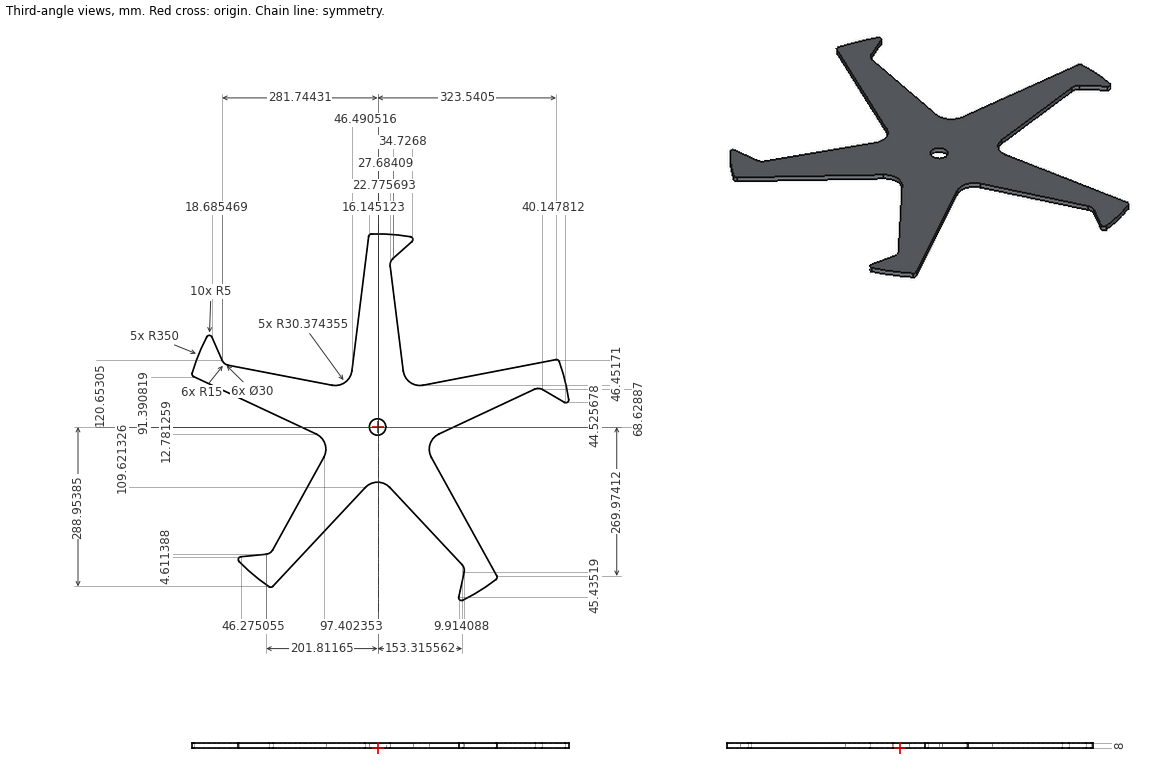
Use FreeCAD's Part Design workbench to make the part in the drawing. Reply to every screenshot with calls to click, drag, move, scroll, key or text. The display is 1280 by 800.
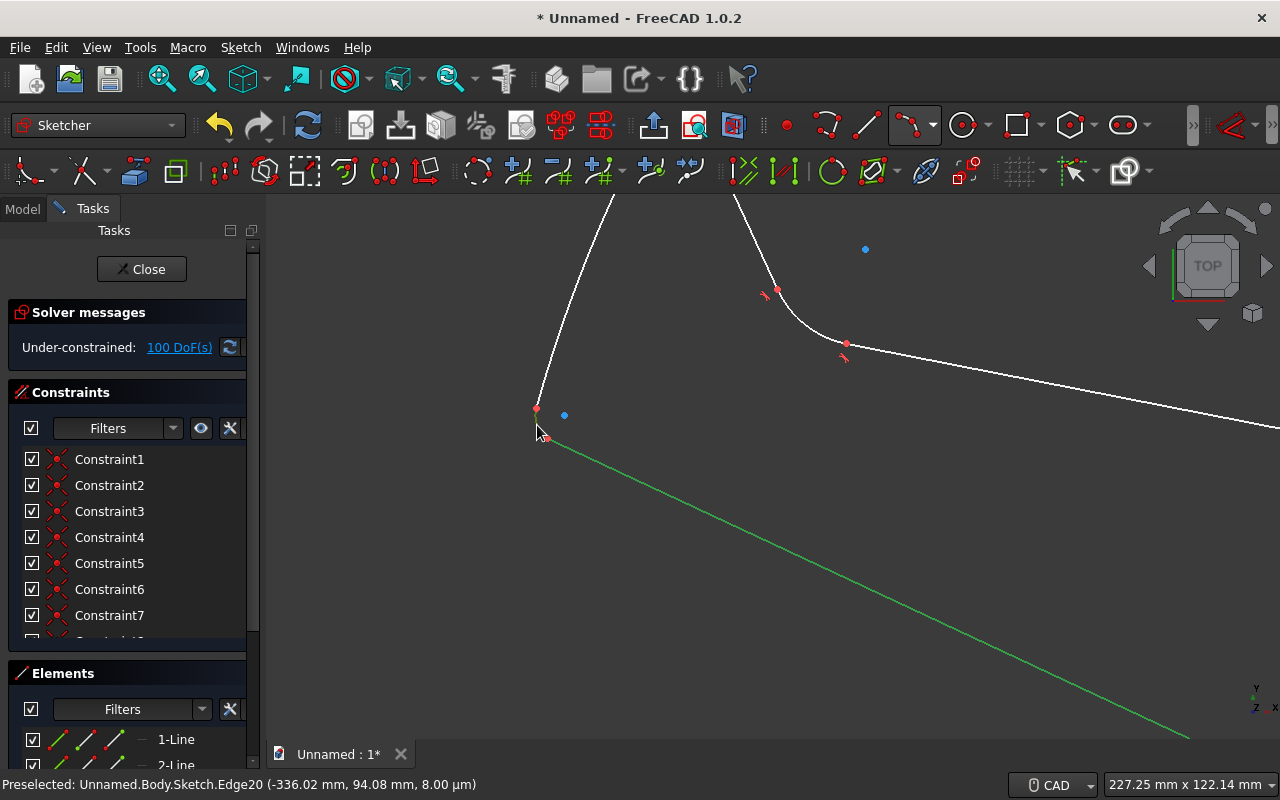
key(t)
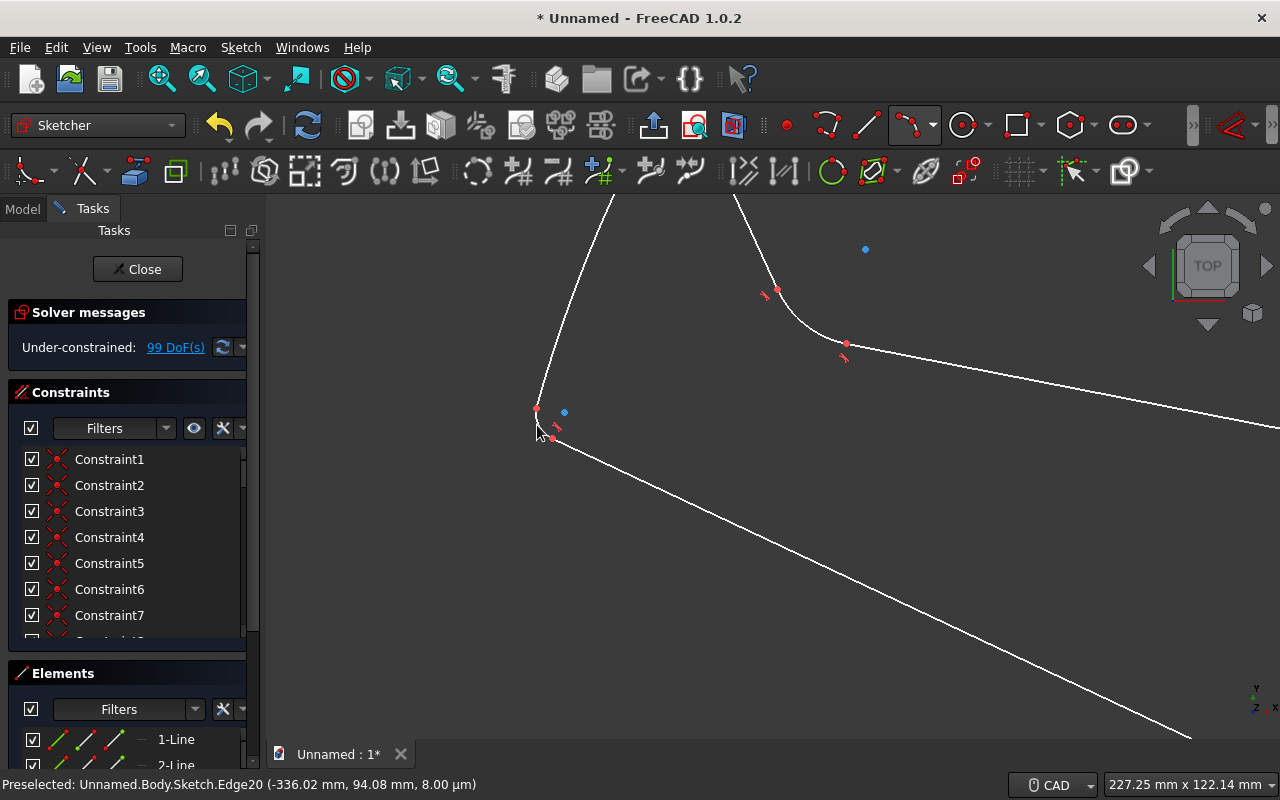
scroll(536, 430, down, 11)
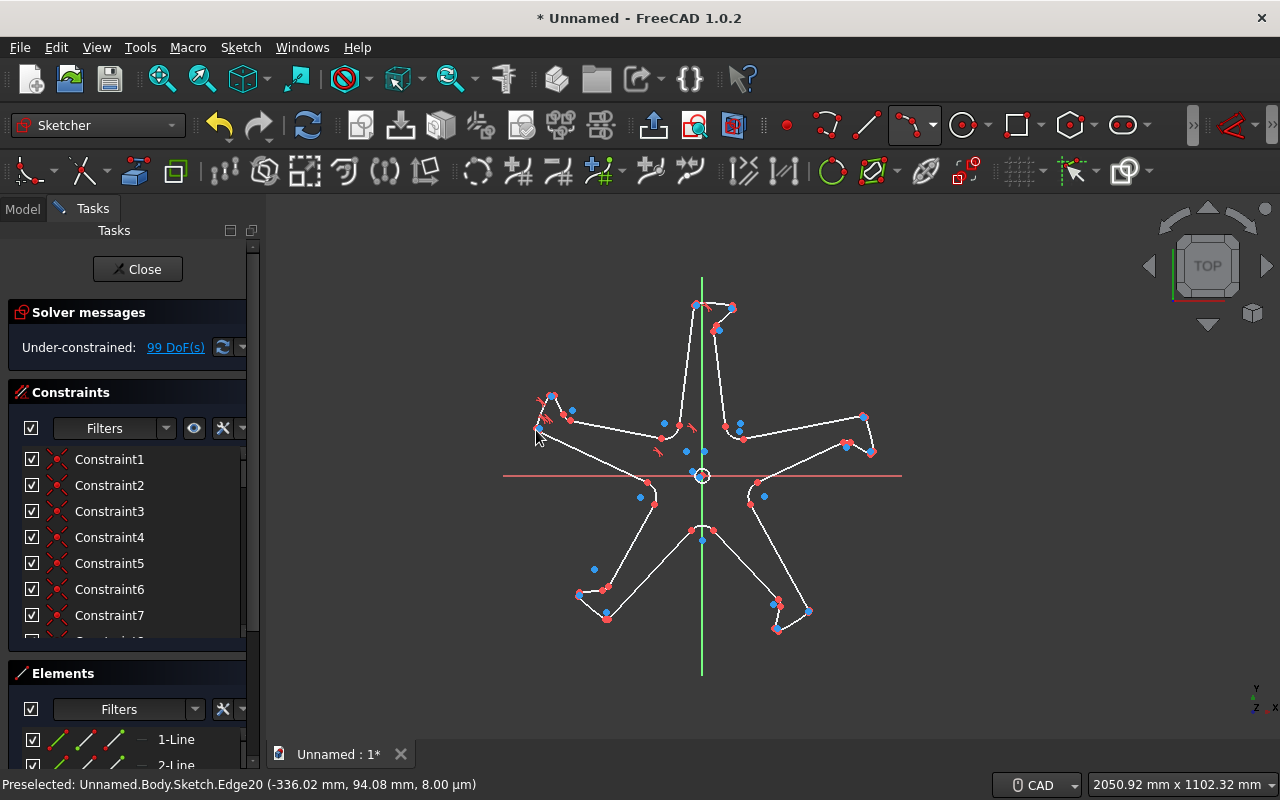
click(571, 447)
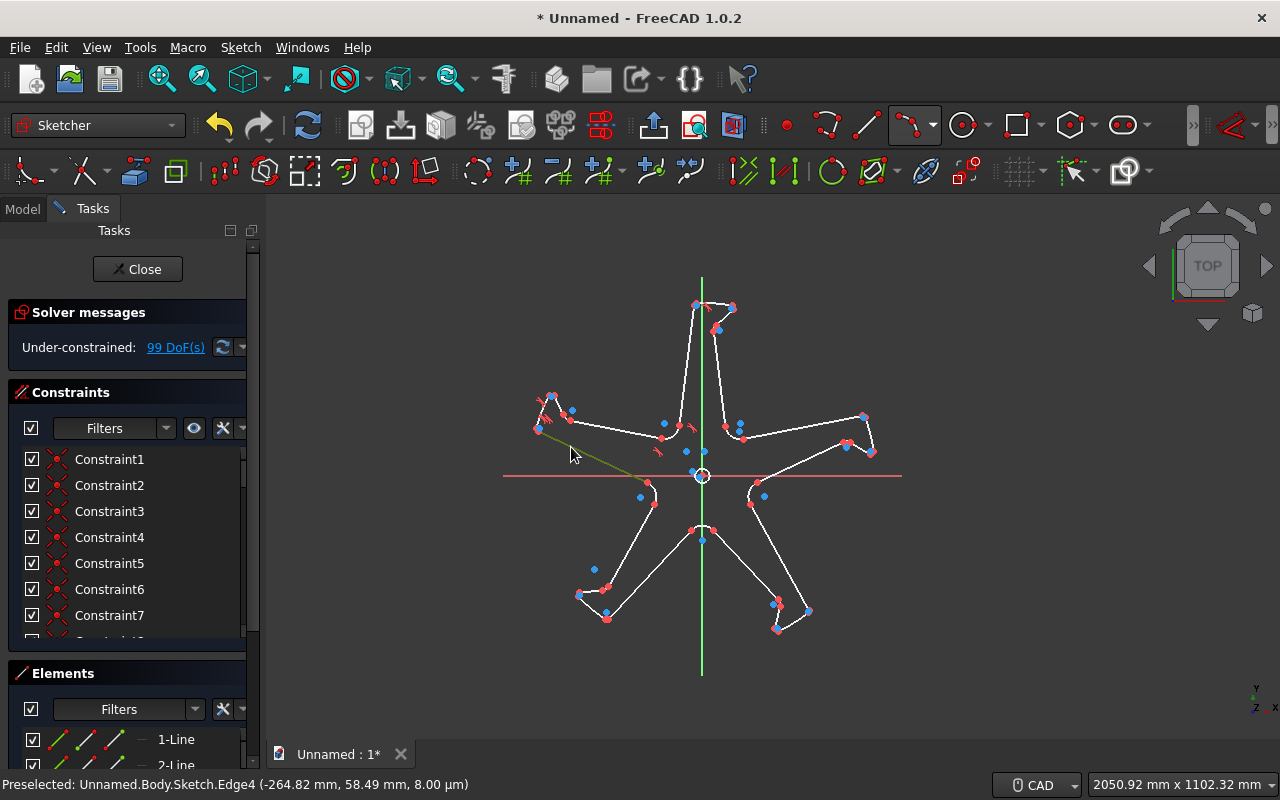
click(656, 492)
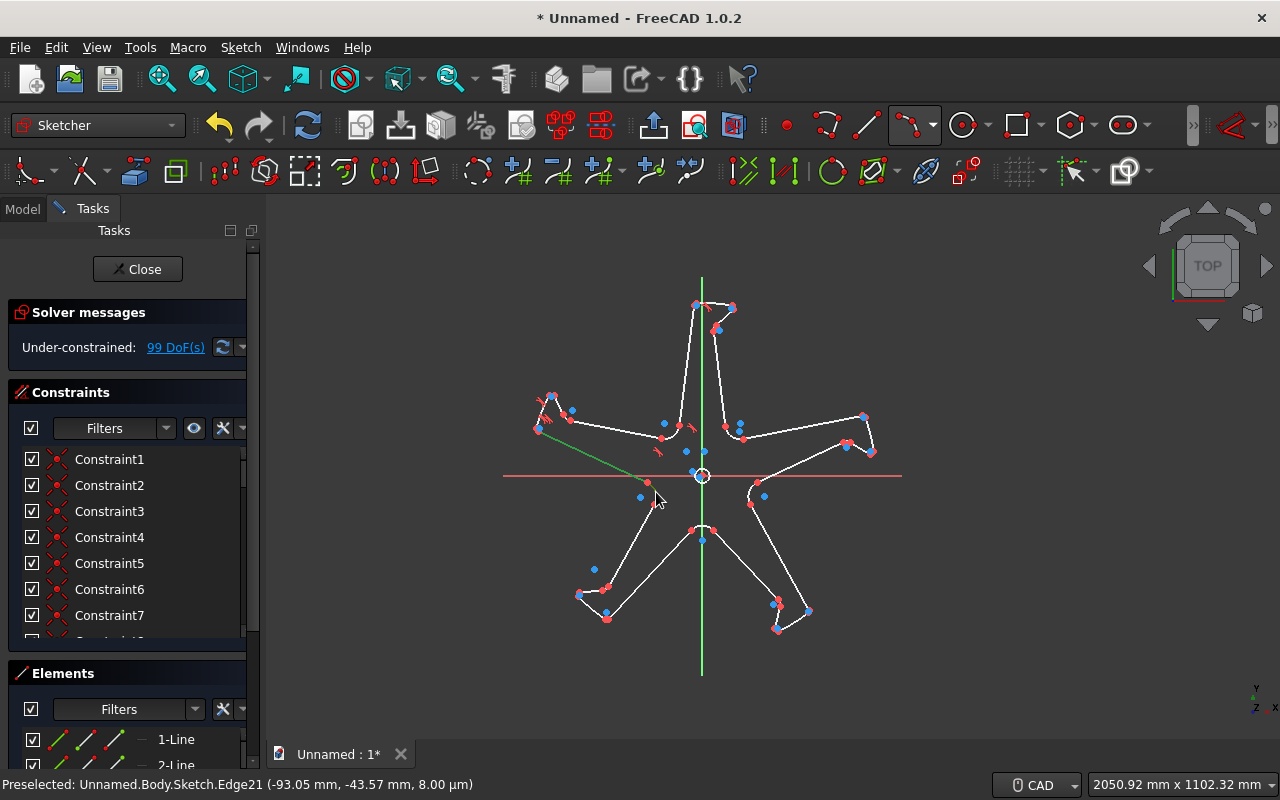
key(t)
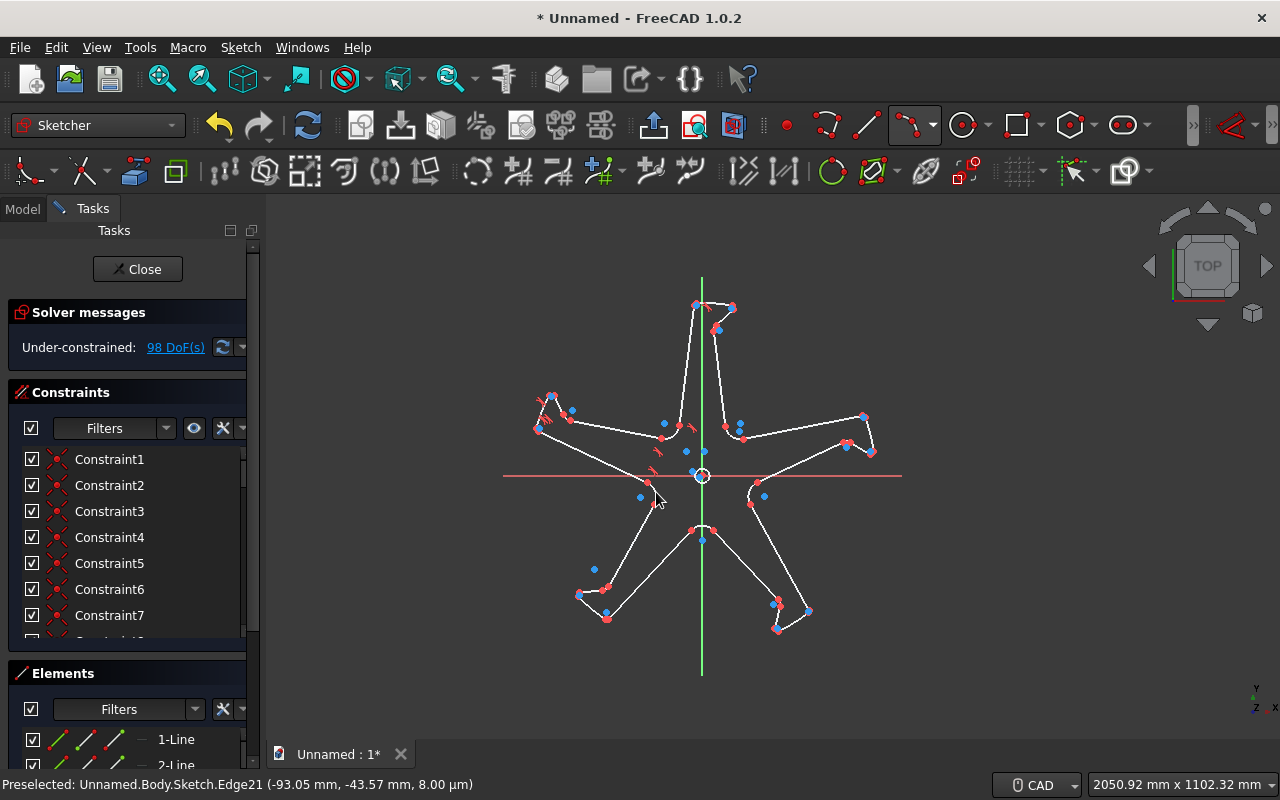
click(641, 529)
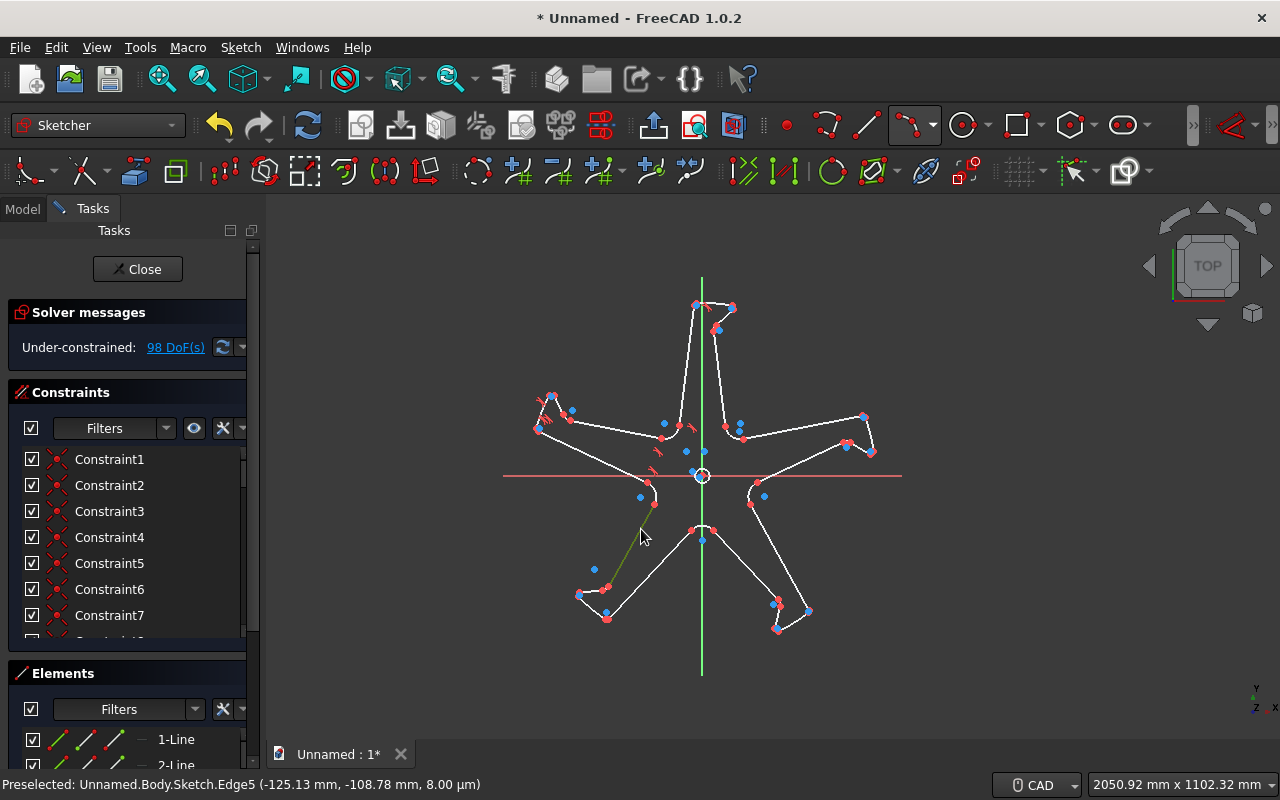
click(655, 492)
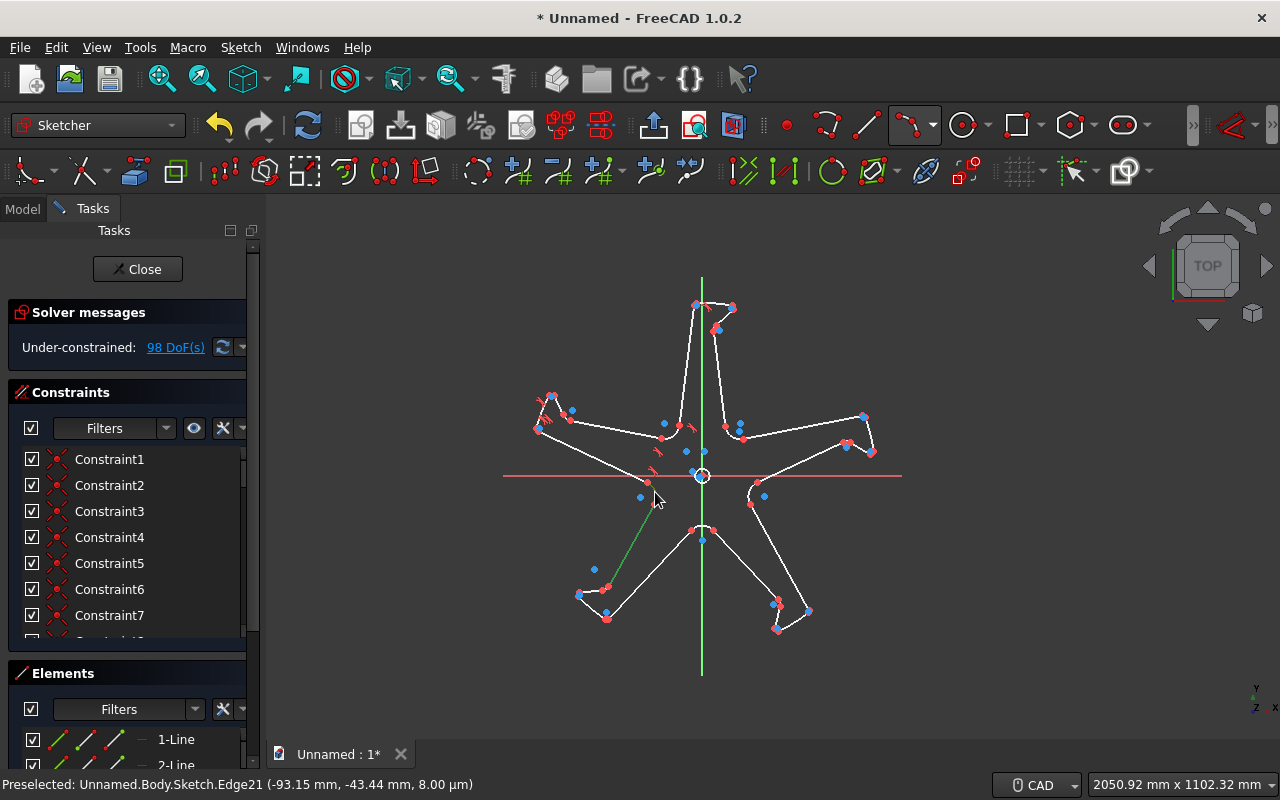
key(t)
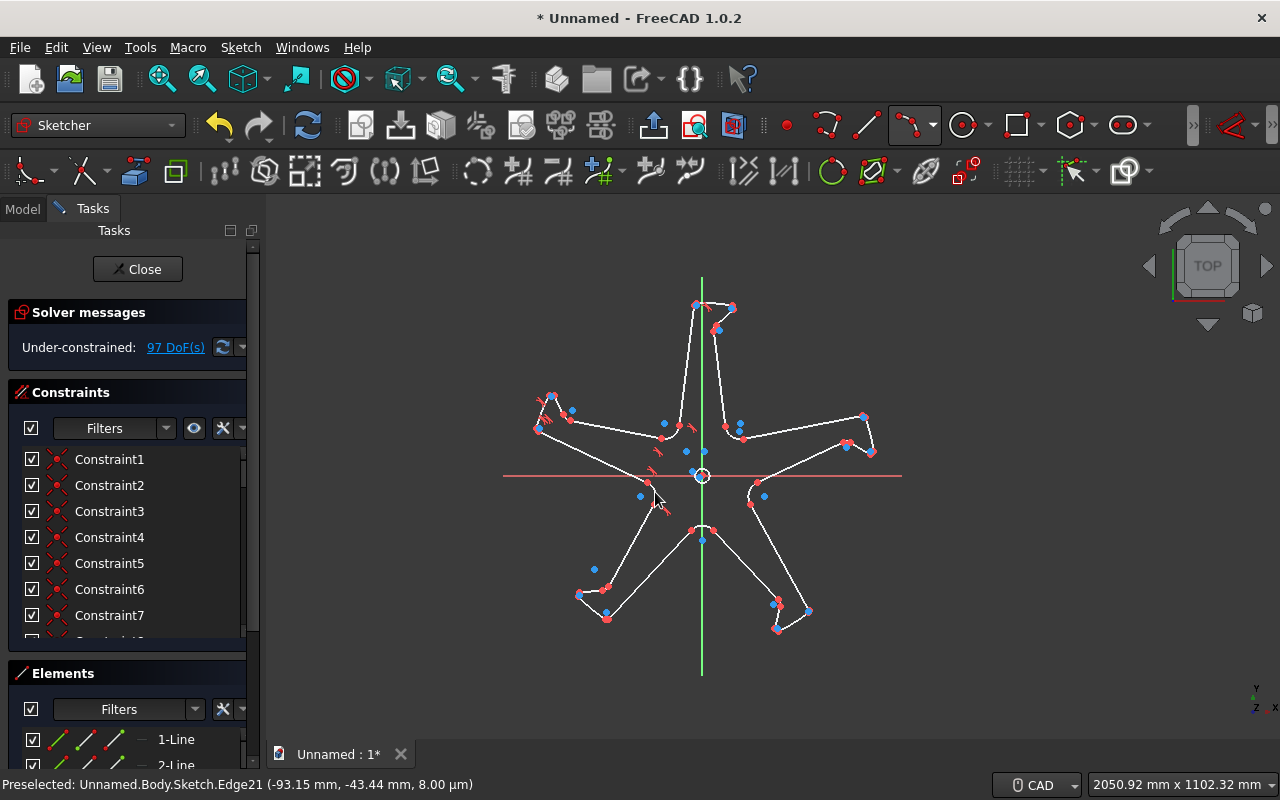
click(640, 529)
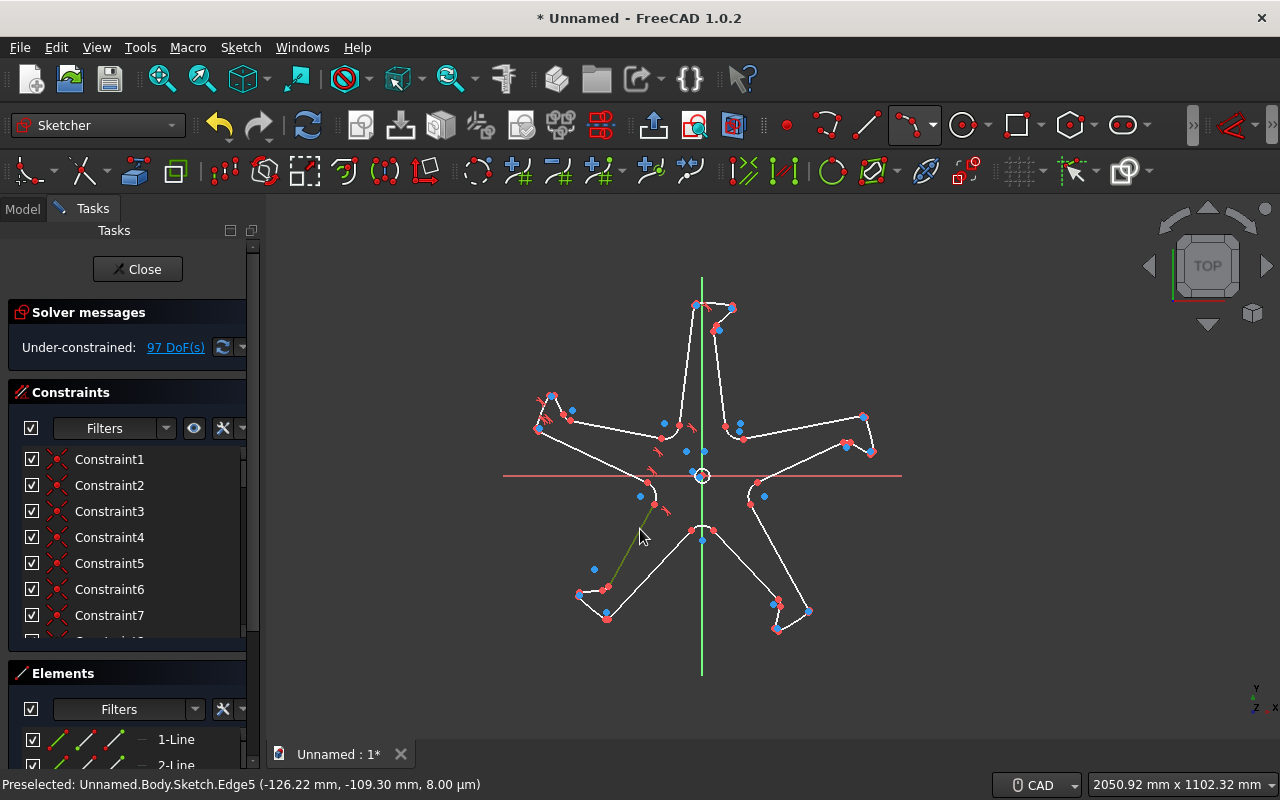
scroll(606, 589, up, 7)